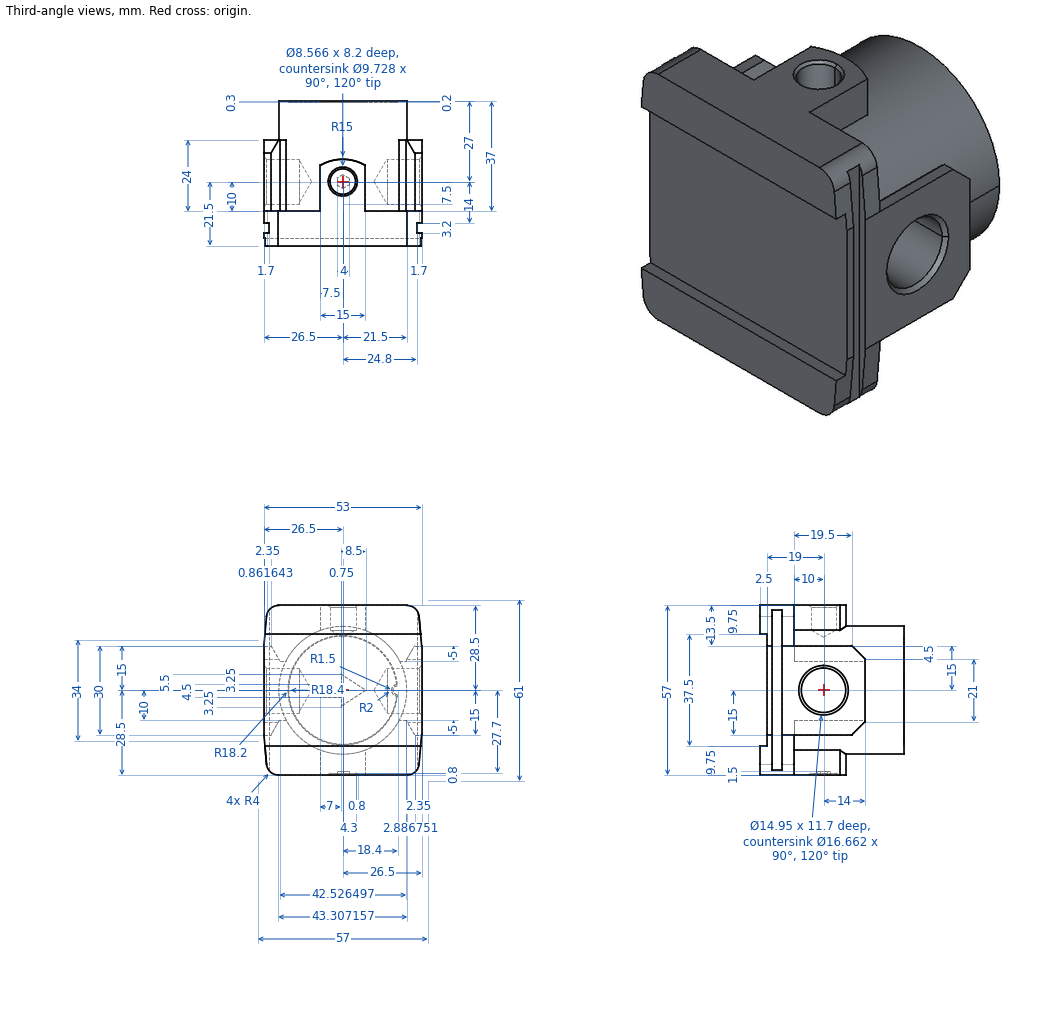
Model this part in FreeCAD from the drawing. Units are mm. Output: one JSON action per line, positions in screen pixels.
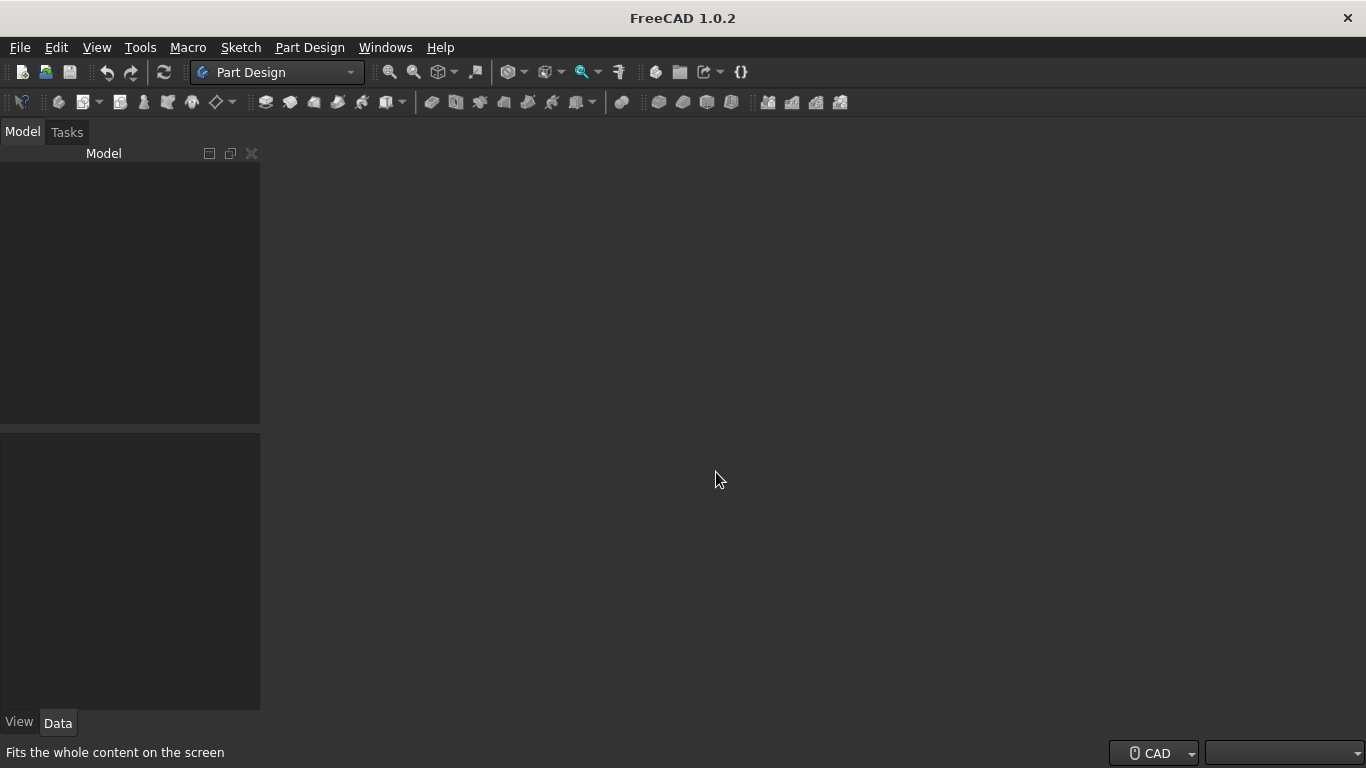
{"action": "left_click", "coordinate": [22, 72]}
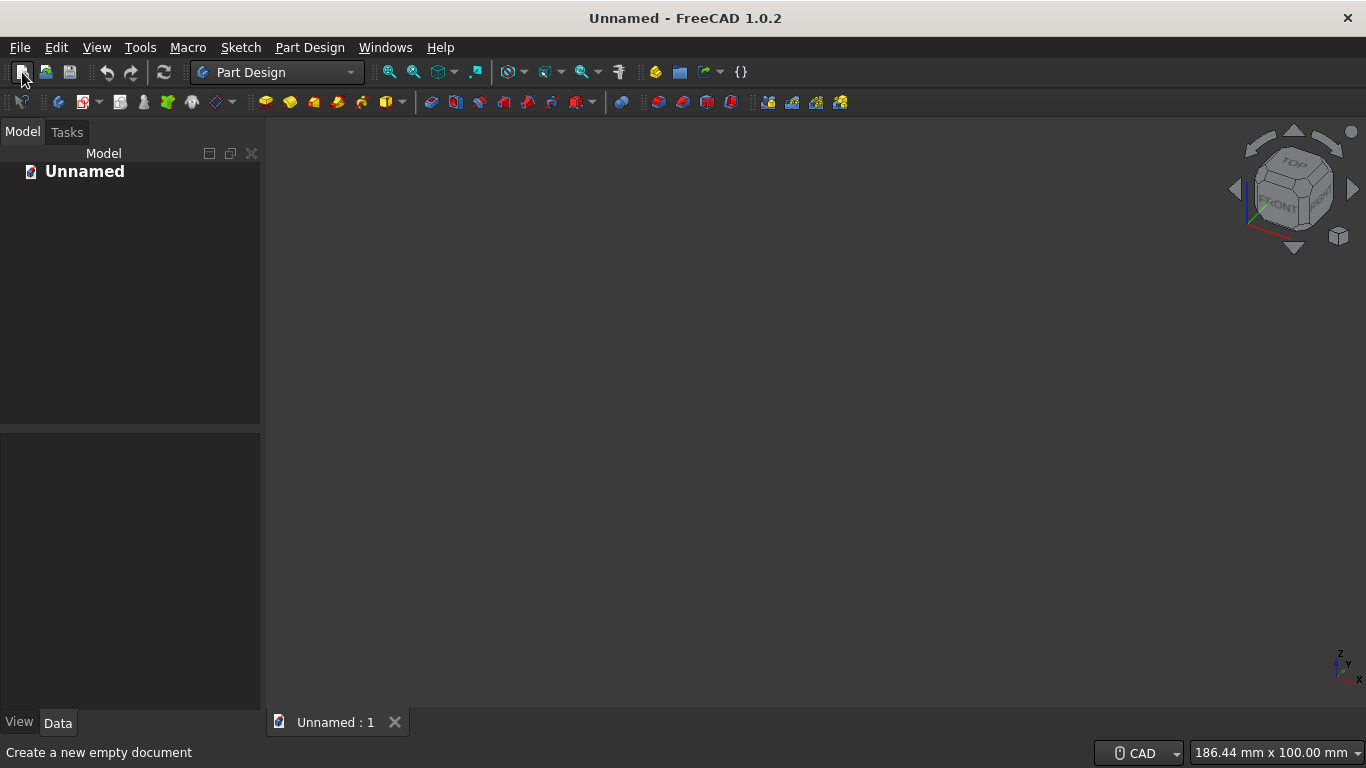
{"action": "left_click", "coordinate": [84, 102]}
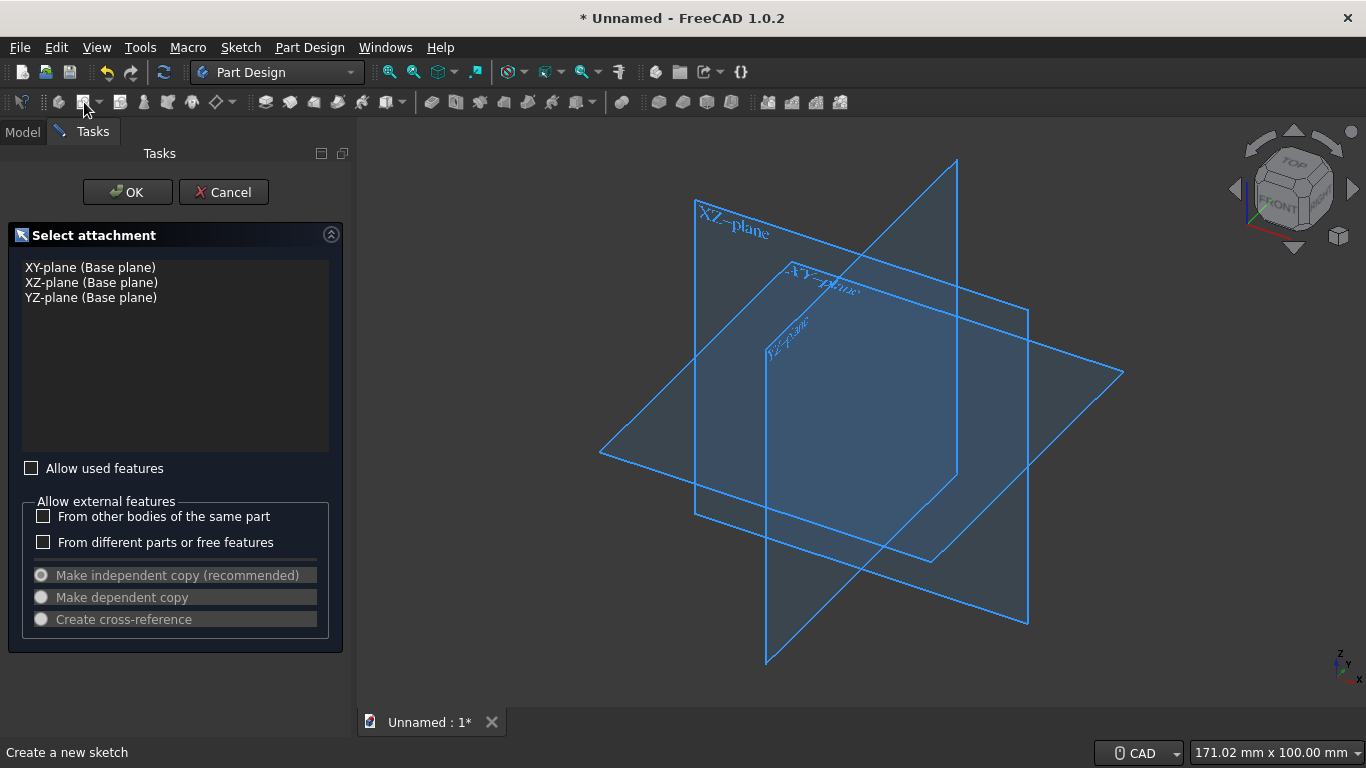
{"action": "left_click", "coordinate": [82, 298]}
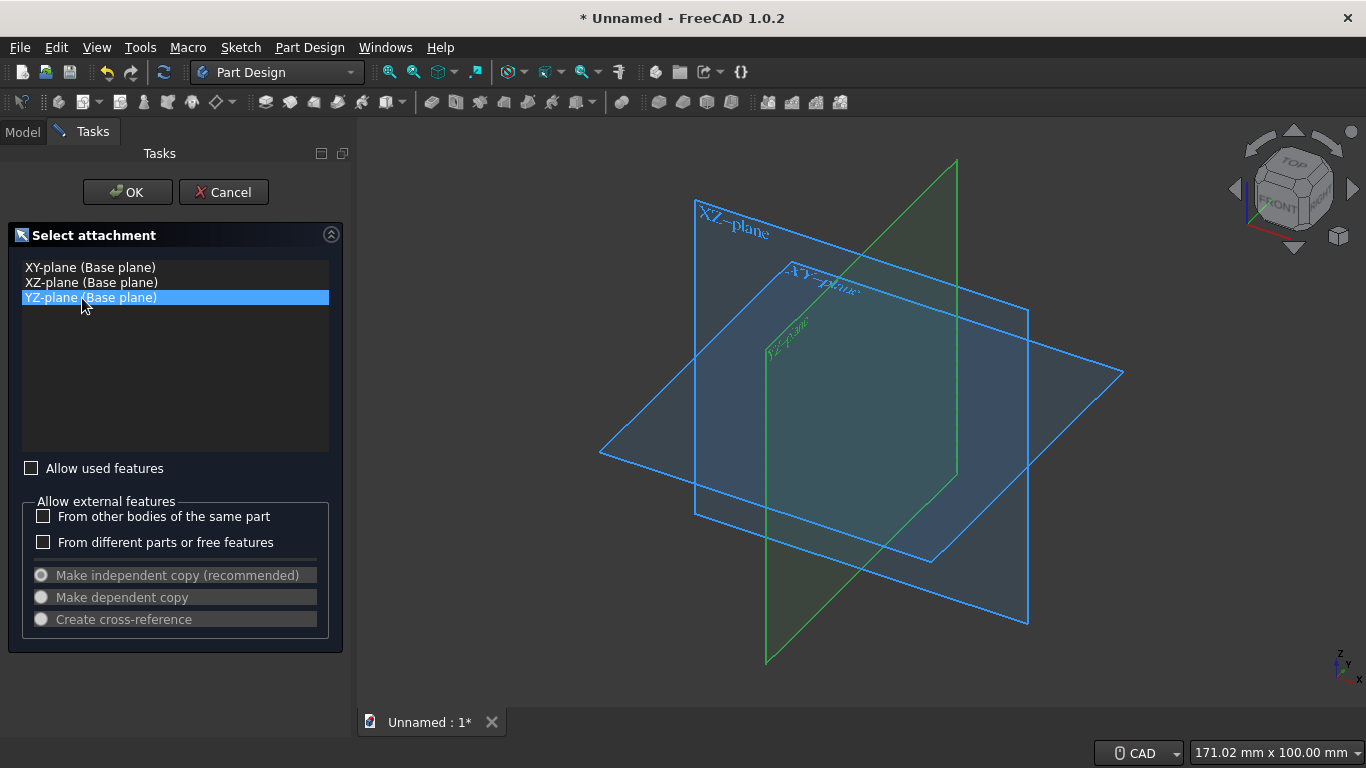
{"action": "left_click", "coordinate": [128, 192]}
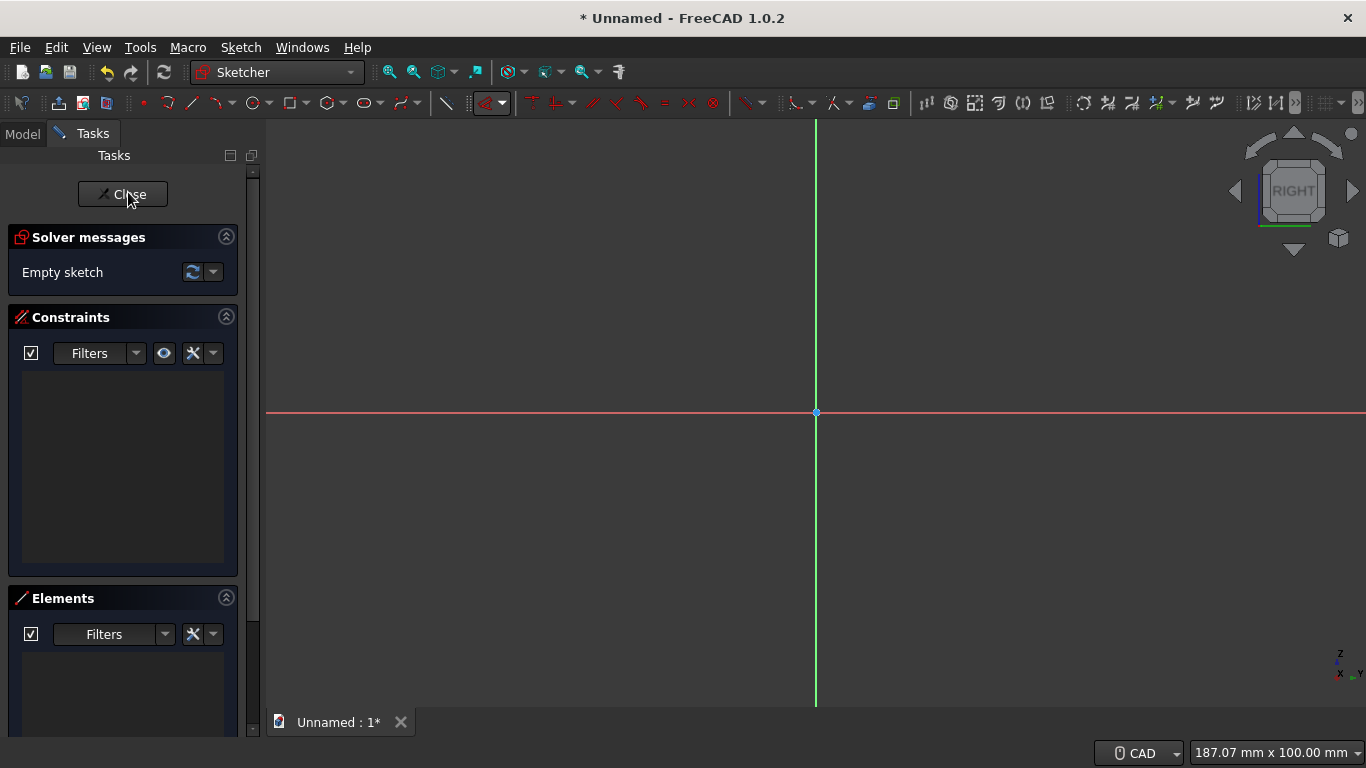
{"action": "left_click", "coordinate": [168, 104]}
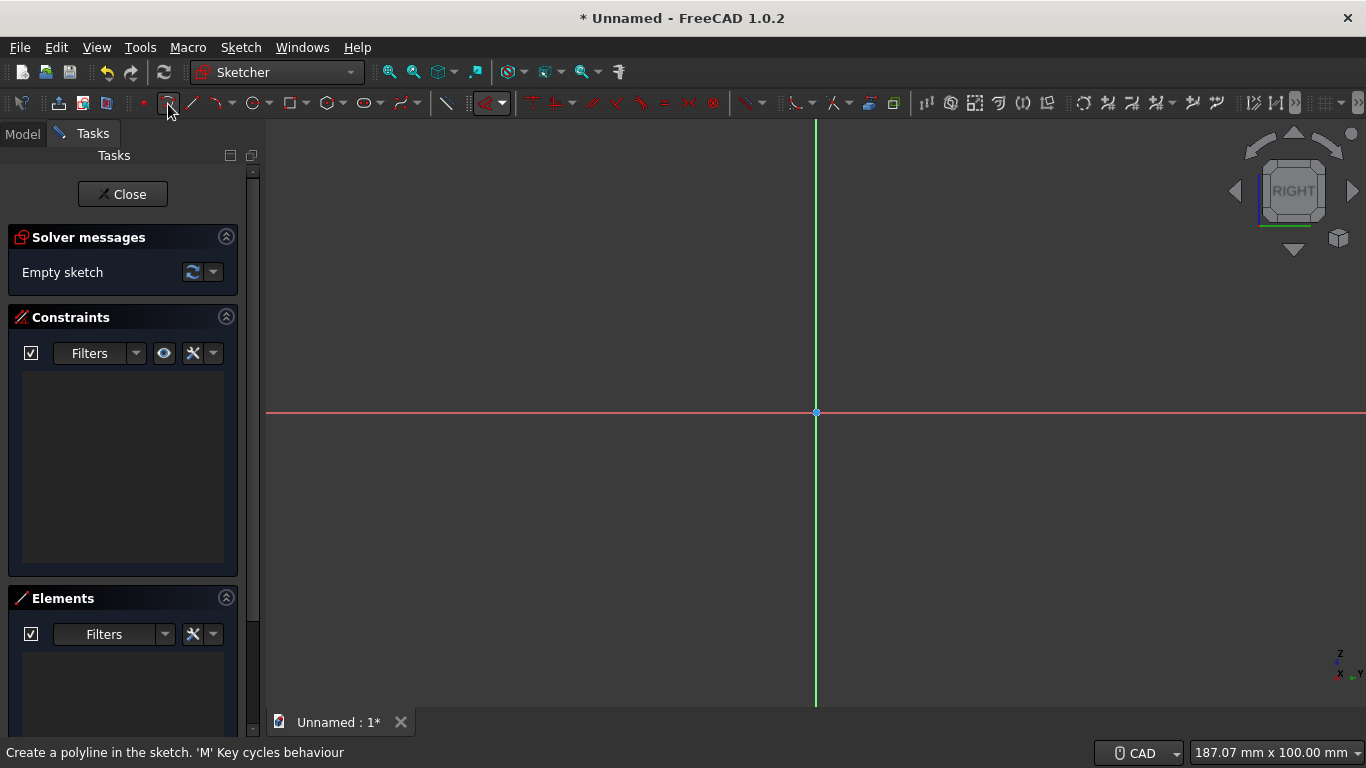
{"action": "left_click", "coordinate": [898, 475]}
{"action": "left_click", "coordinate": [898, 351]}
{"action": "left_click", "coordinate": [872, 325]}
{"action": "left_click", "coordinate": [757, 325]}
{"action": "left_click", "coordinate": [757, 245]}
{"action": "left_click", "coordinate": [690, 245]}
{"action": "left_click", "coordinate": [690, 303]}
{"action": "left_click", "coordinate": [704, 303]}
{"action": "left_click", "coordinate": [704, 523]}
{"action": "left_click", "coordinate": [690, 523]}
{"action": "left_click", "coordinate": [690, 581]}
{"action": "left_click", "coordinate": [757, 581]}
{"action": "left_click", "coordinate": [757, 501]}
{"action": "left_click", "coordinate": [872, 501]}
{"action": "left_click", "coordinate": [898, 476]}
{"action": "key", "text": "Escape"}
{"action": "key", "text": "Escape"}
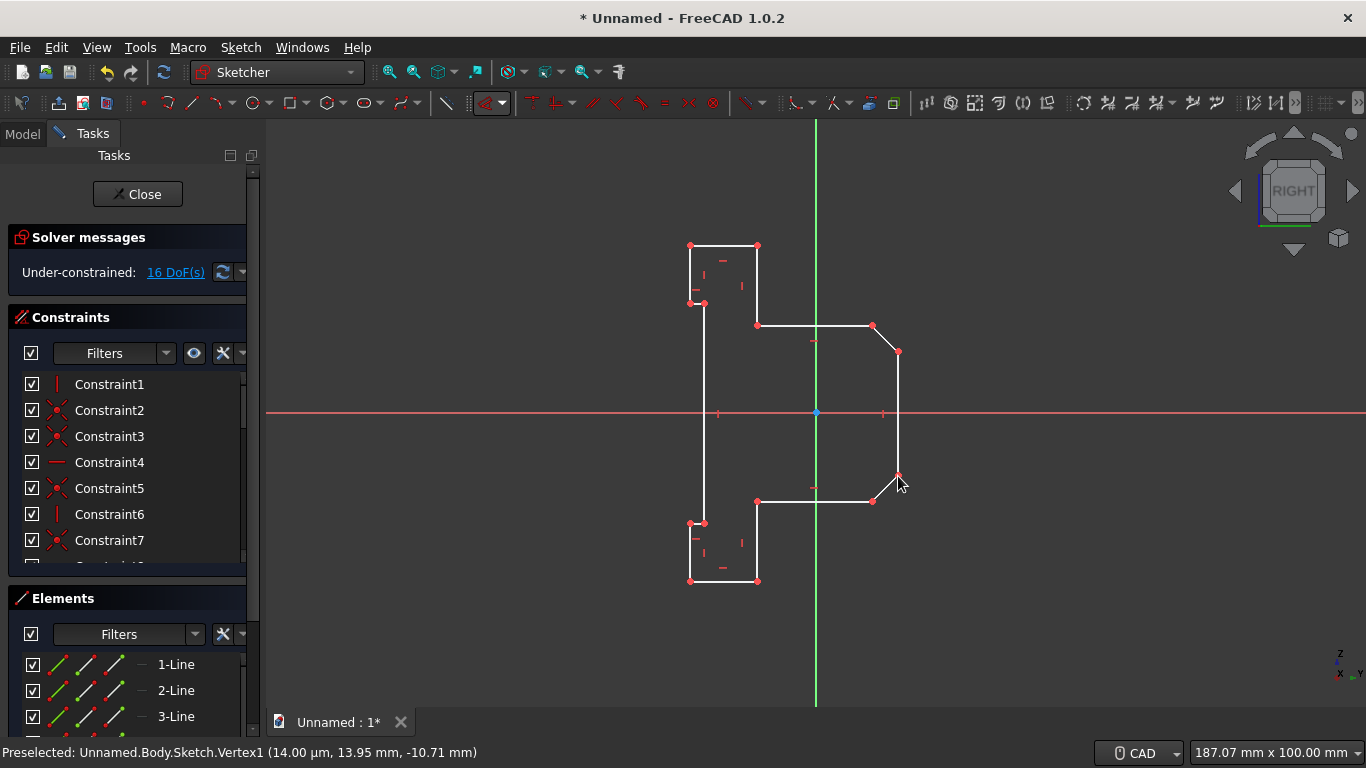
{"action": "left_click", "coordinate": [486, 104]}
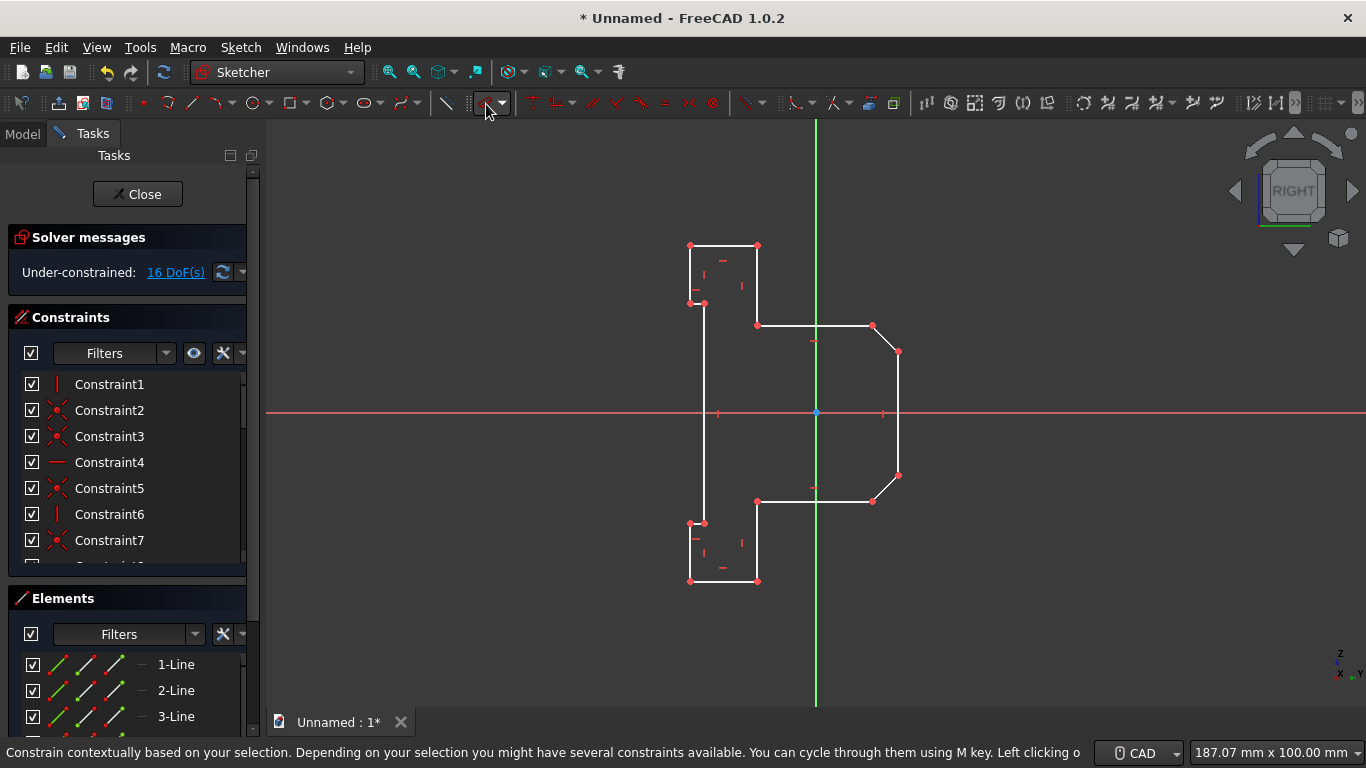
{"action": "left_click", "coordinate": [898, 439]}
{"action": "left_click", "coordinate": [932, 385]}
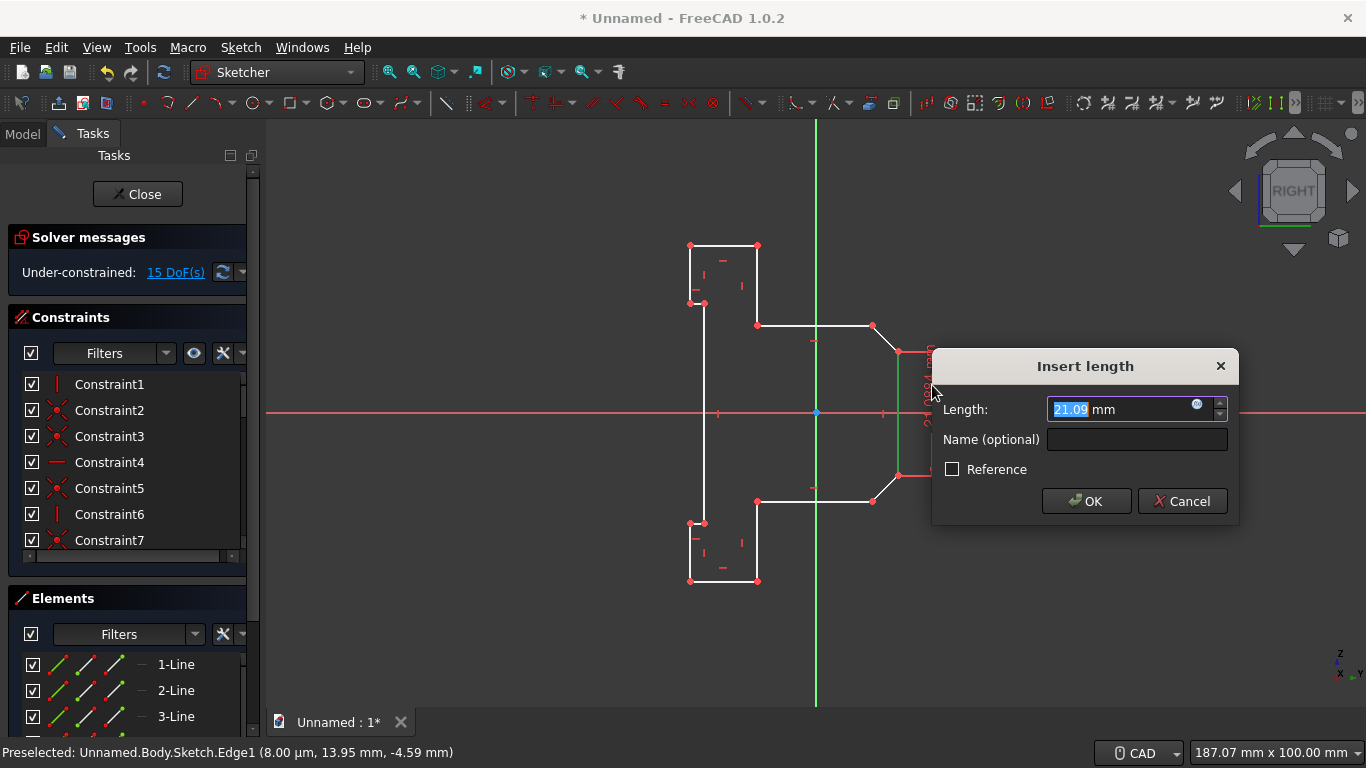
{"action": "type", "text": "21"}
{"action": "key", "text": "Return"}